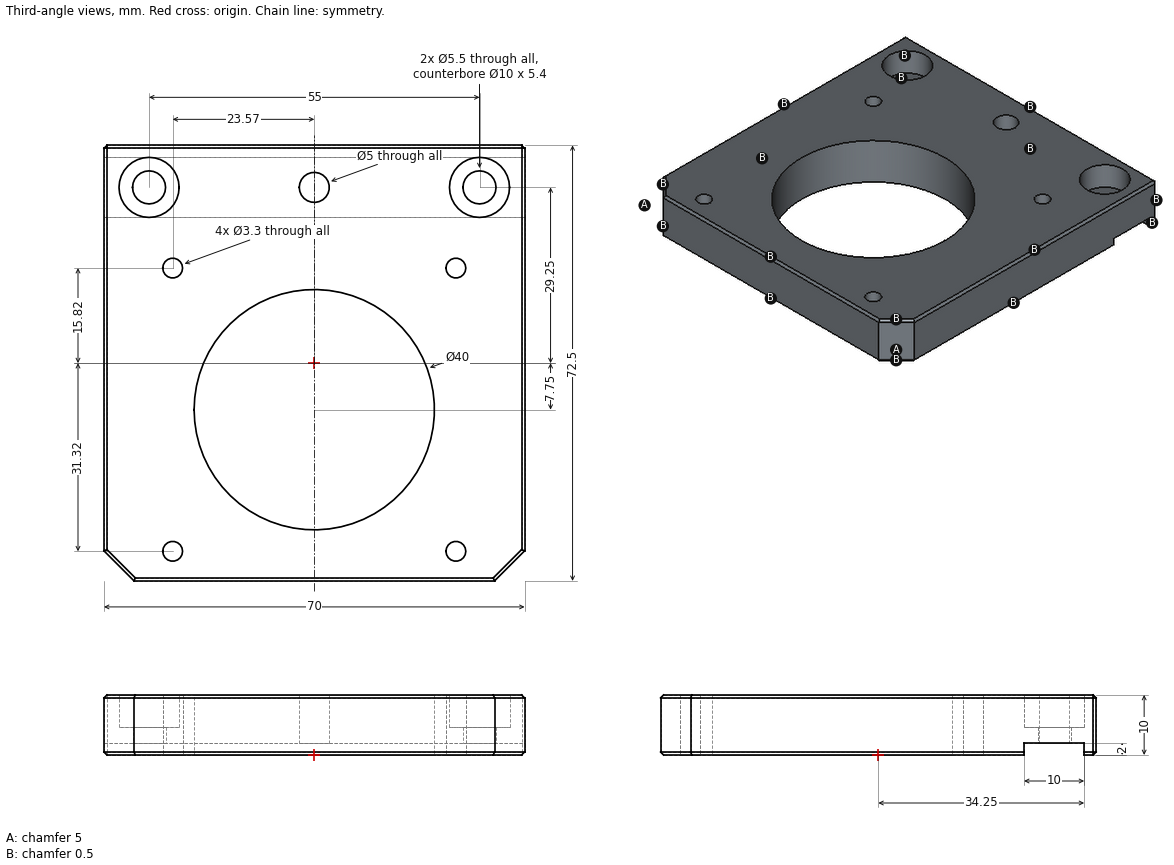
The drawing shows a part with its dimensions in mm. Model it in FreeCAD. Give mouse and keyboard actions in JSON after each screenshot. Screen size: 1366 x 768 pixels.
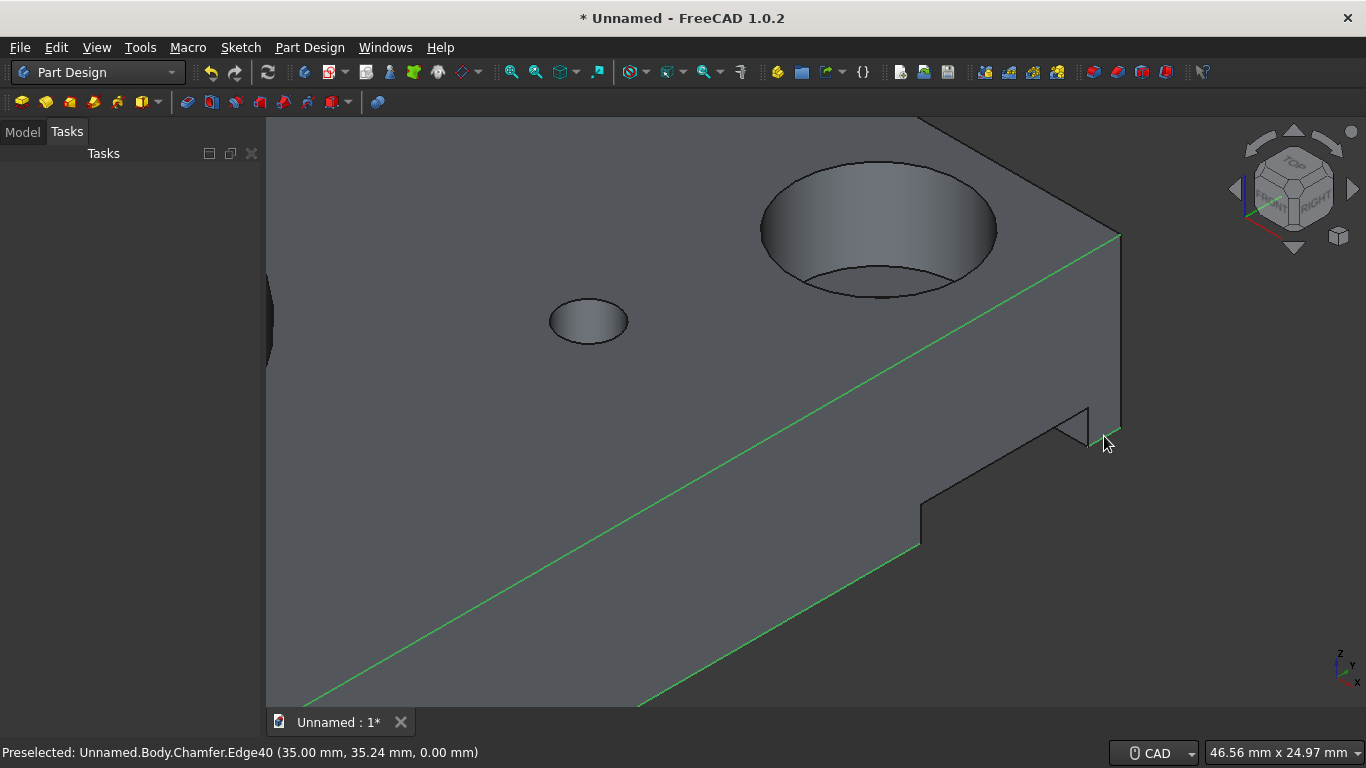
{"action": "left_click", "coordinate": [1118, 72]}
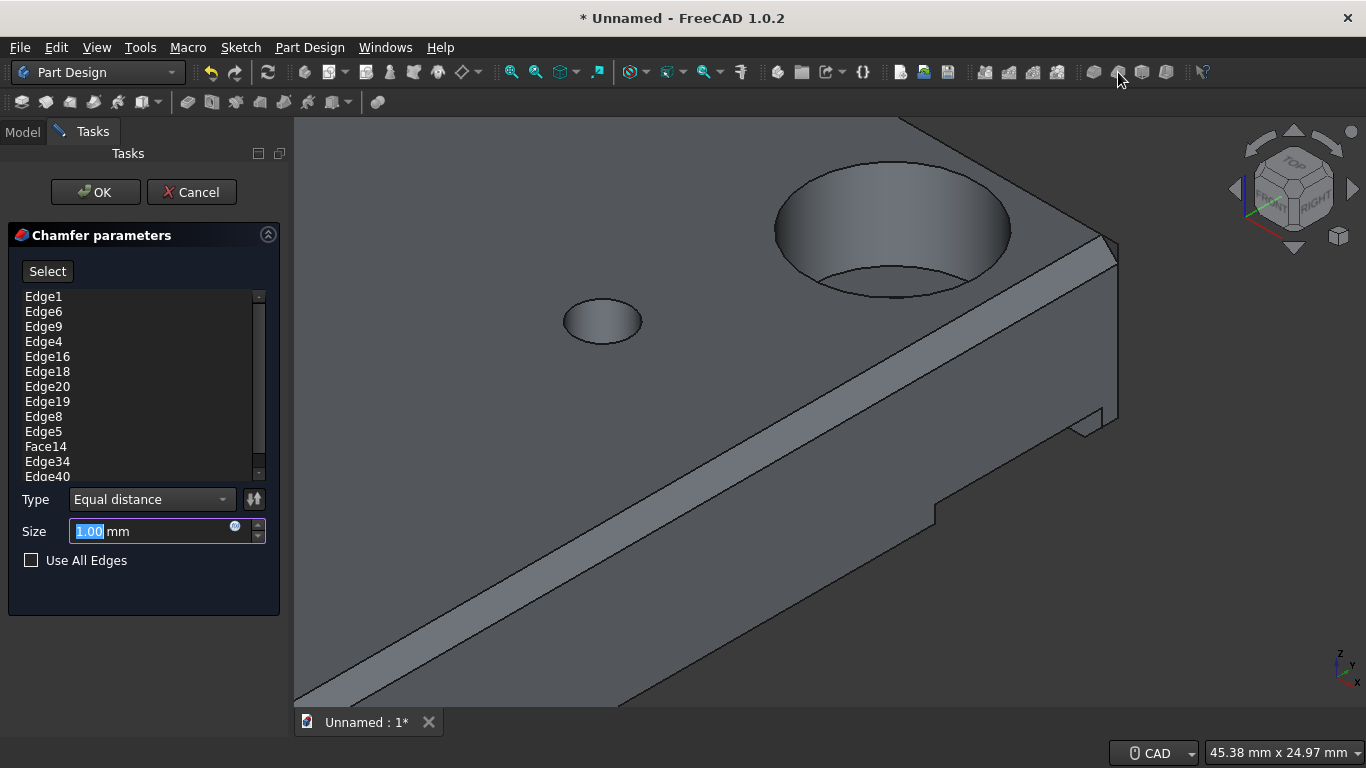
{"action": "type", "text": "0.5"}
{"action": "key", "text": "Tab"}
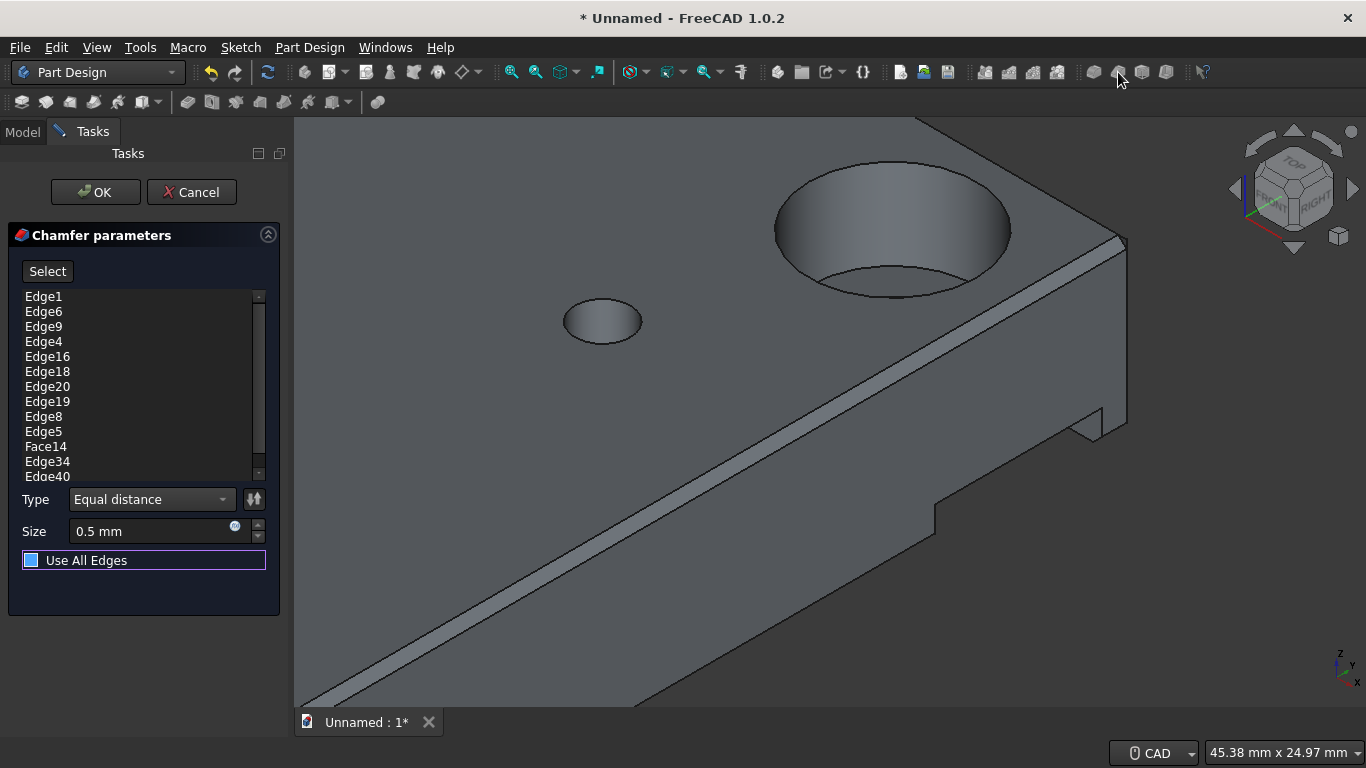
{"action": "left_click", "coordinate": [96, 192]}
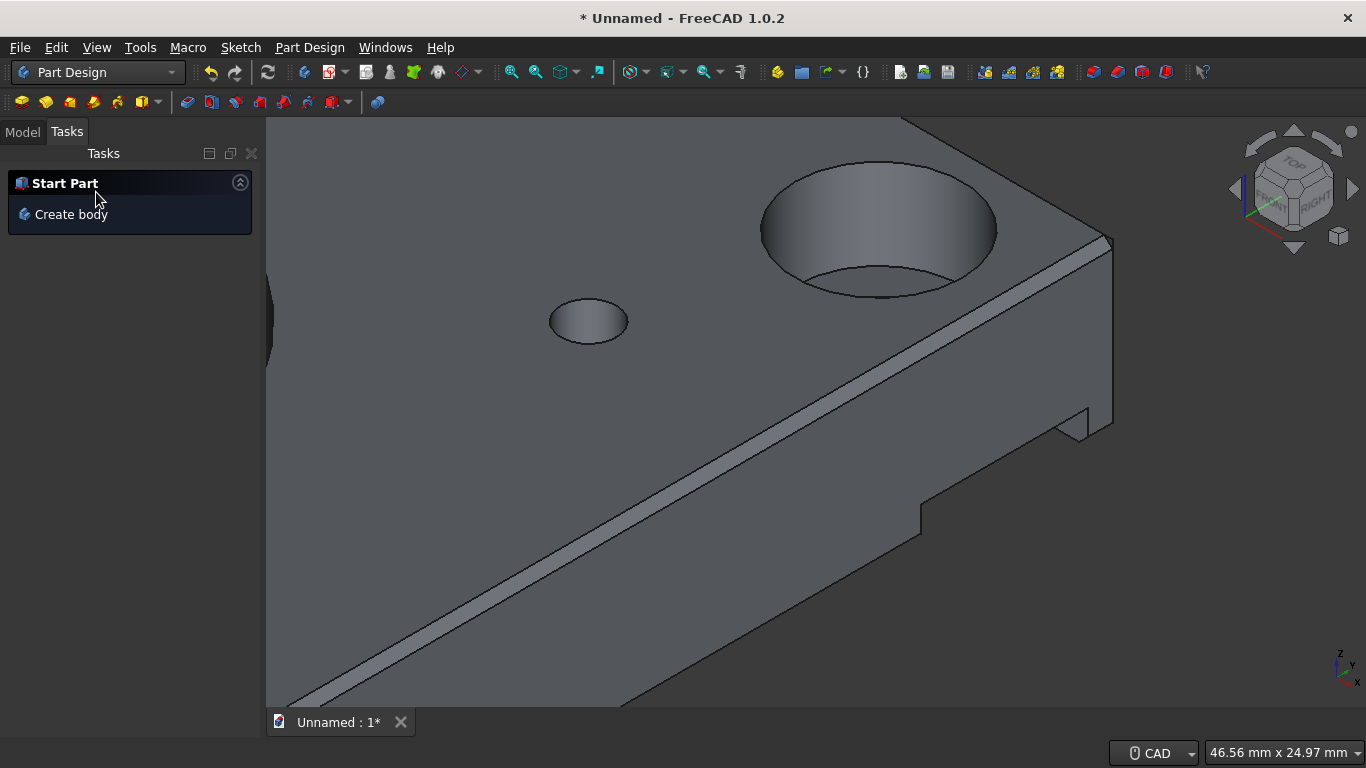
{"action": "left_click", "coordinate": [512, 72]}